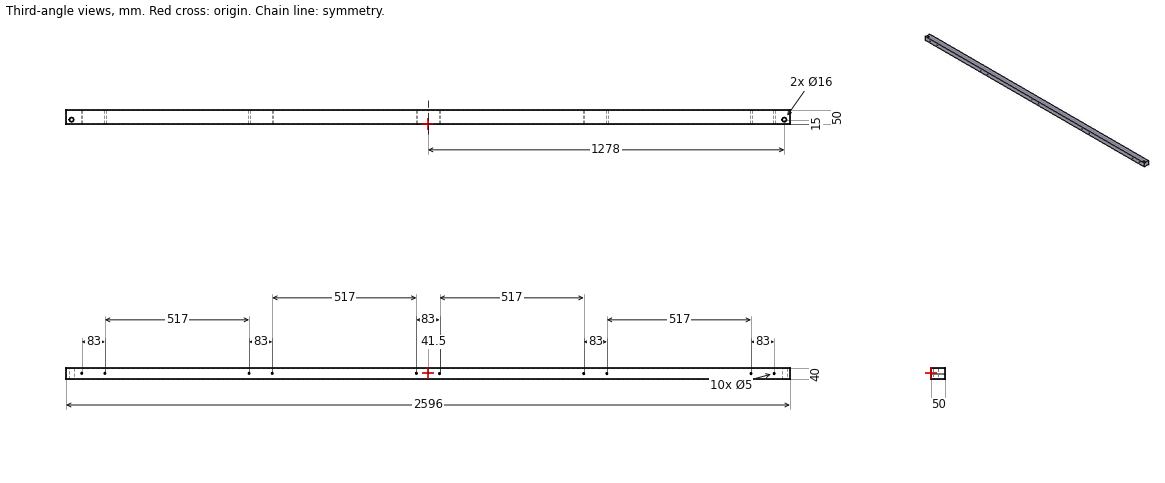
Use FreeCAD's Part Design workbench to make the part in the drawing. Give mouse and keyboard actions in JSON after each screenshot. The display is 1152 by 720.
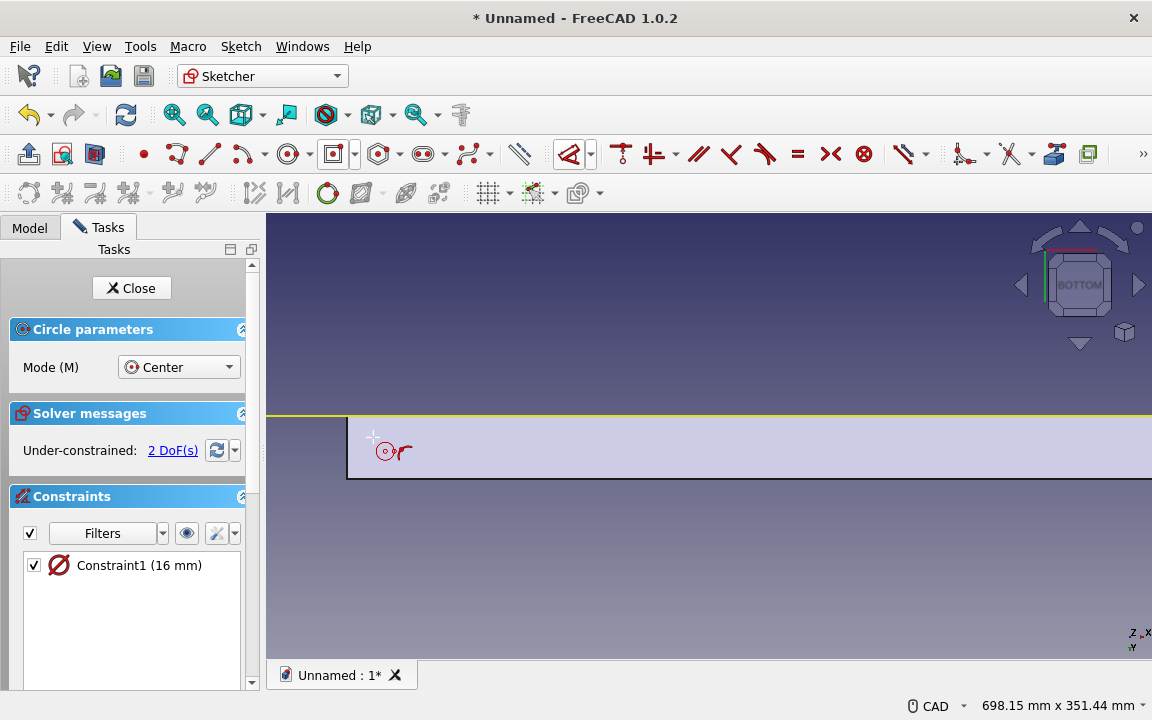
{"action": "left_click", "coordinate": [372, 435]}
{"action": "mouse_move", "coordinate": [379, 442]}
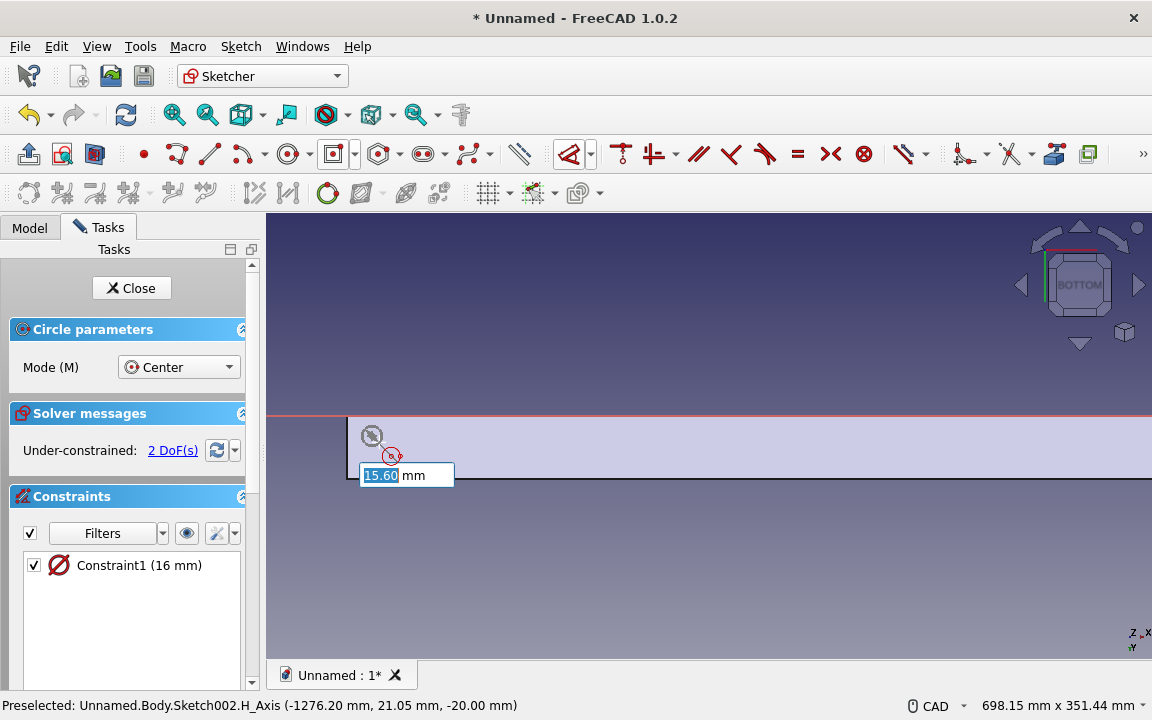
{"action": "type", "text": "16"}
{"action": "key", "text": "Return"}
{"action": "key", "text": "Escape"}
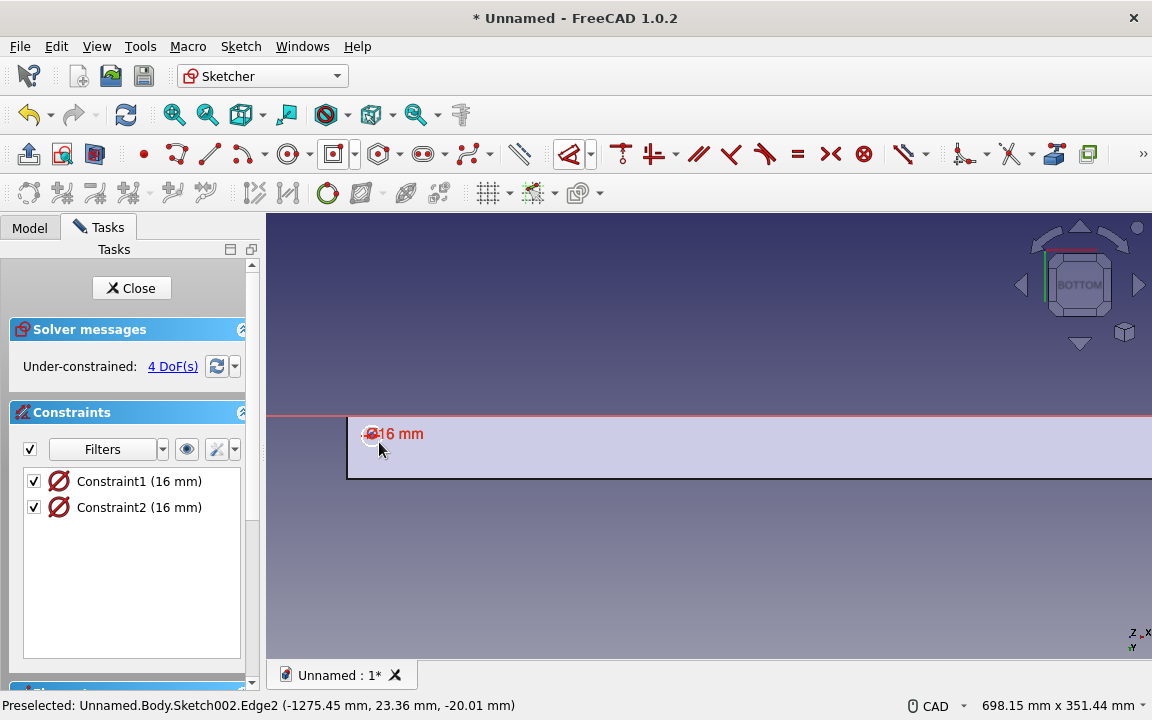
{"action": "scroll", "coordinate": [373, 437], "scroll_direction": "down", "scroll_amount": 9}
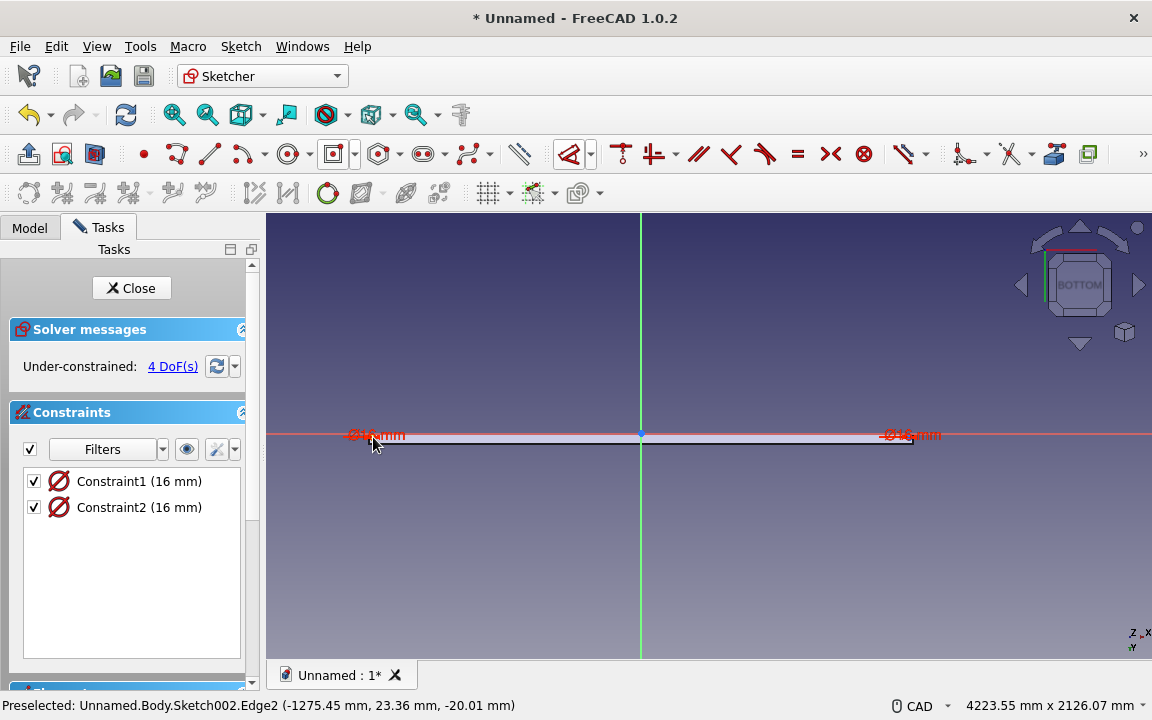
{"action": "left_click", "coordinate": [909, 437]}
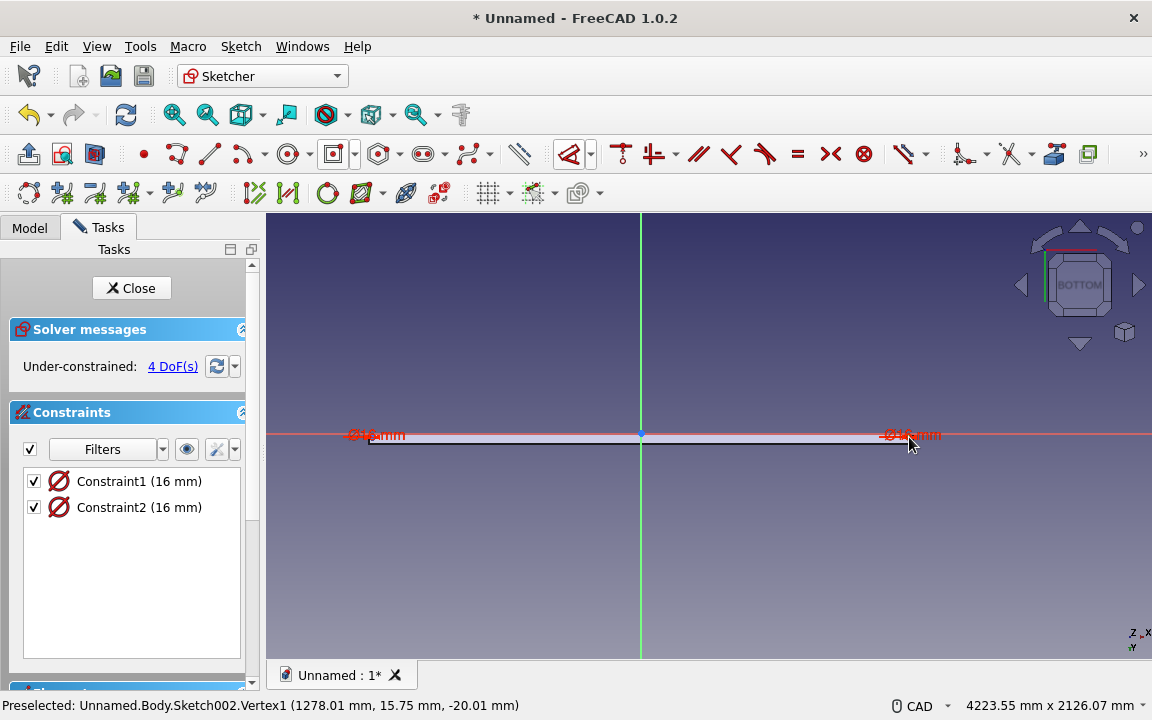
{"action": "left_click", "coordinate": [373, 437]}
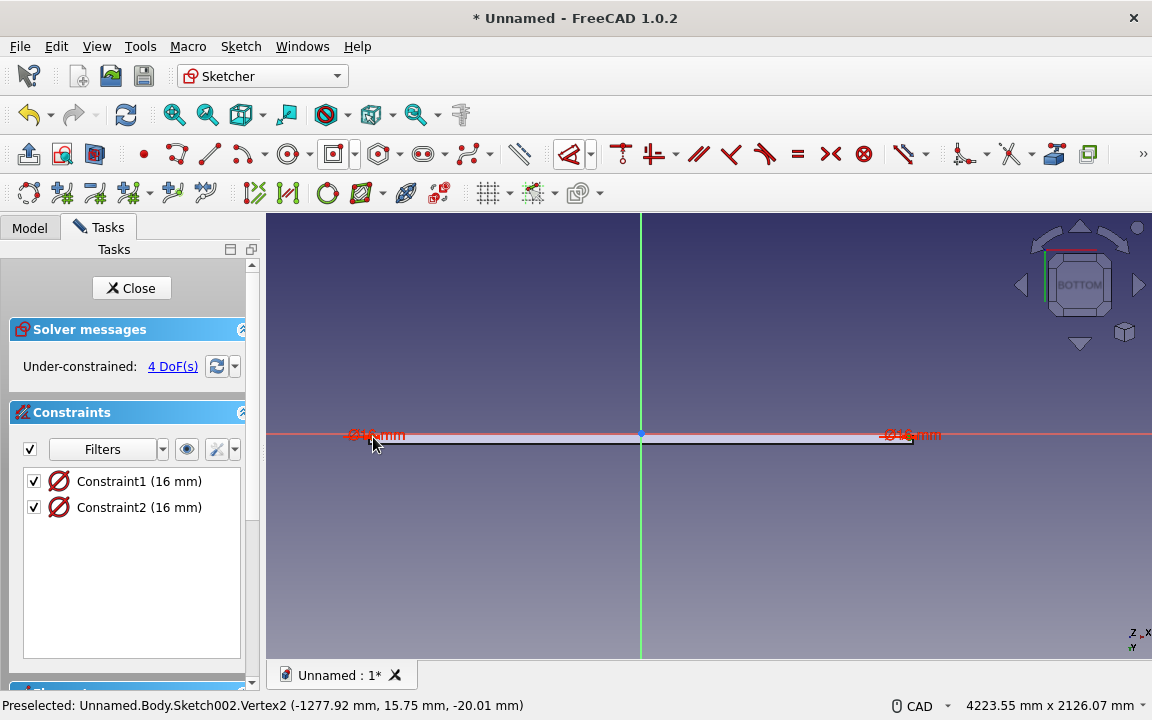
{"action": "left_click", "coordinate": [641, 603]}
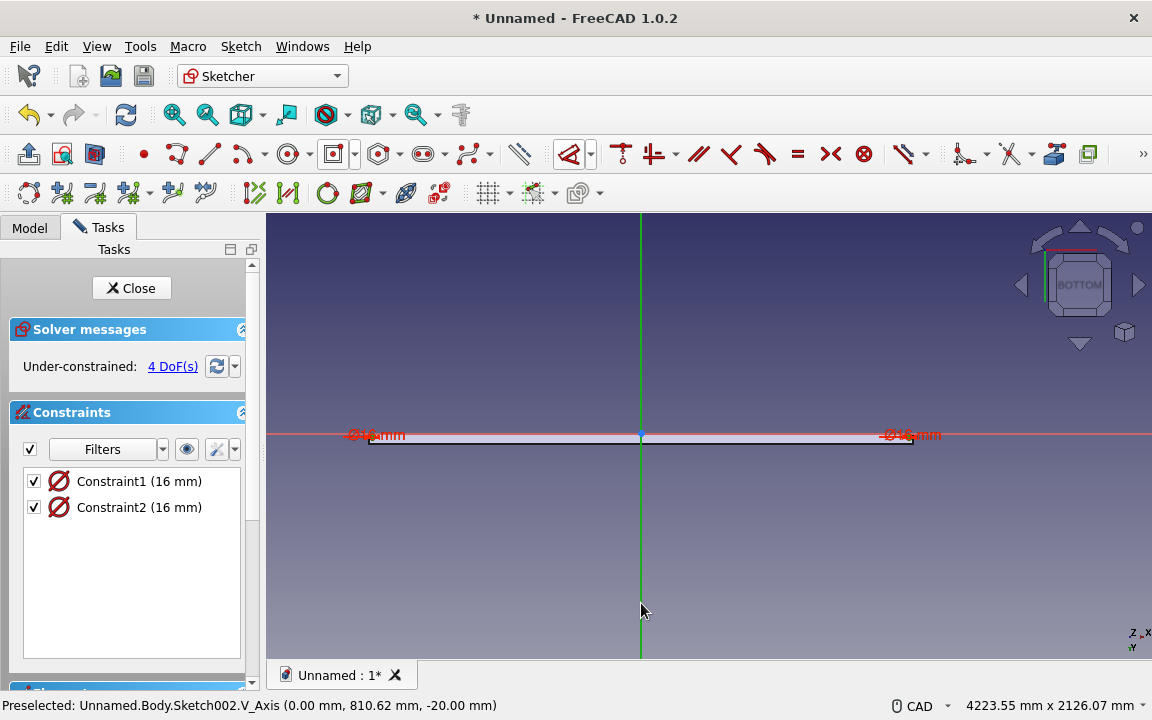
{"action": "left_click", "coordinate": [831, 154]}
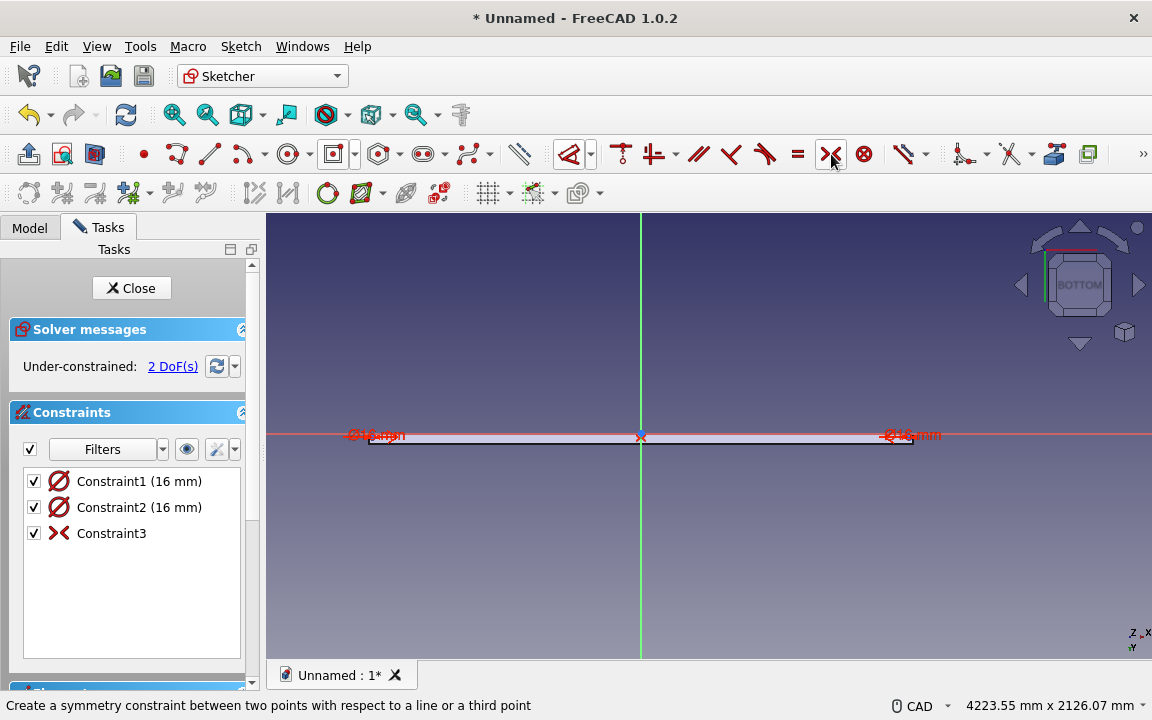
{"action": "scroll", "coordinate": [909, 437], "scroll_direction": "up", "scroll_amount": 13}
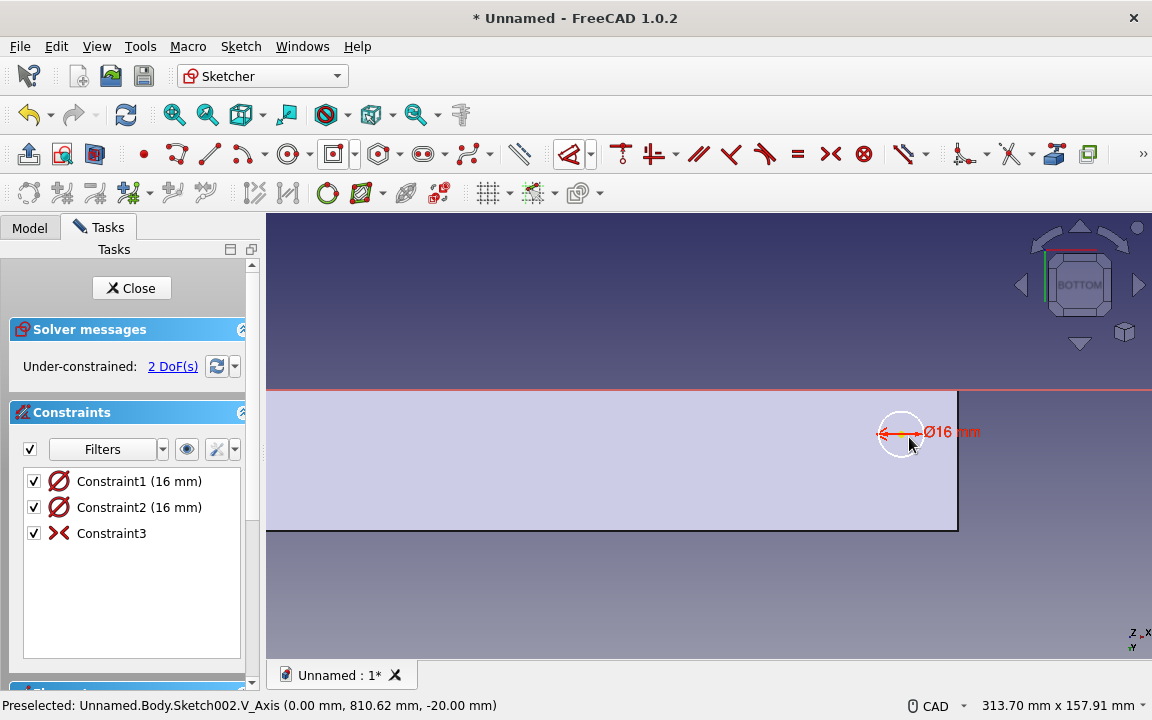
{"action": "left_click", "coordinate": [901, 434]}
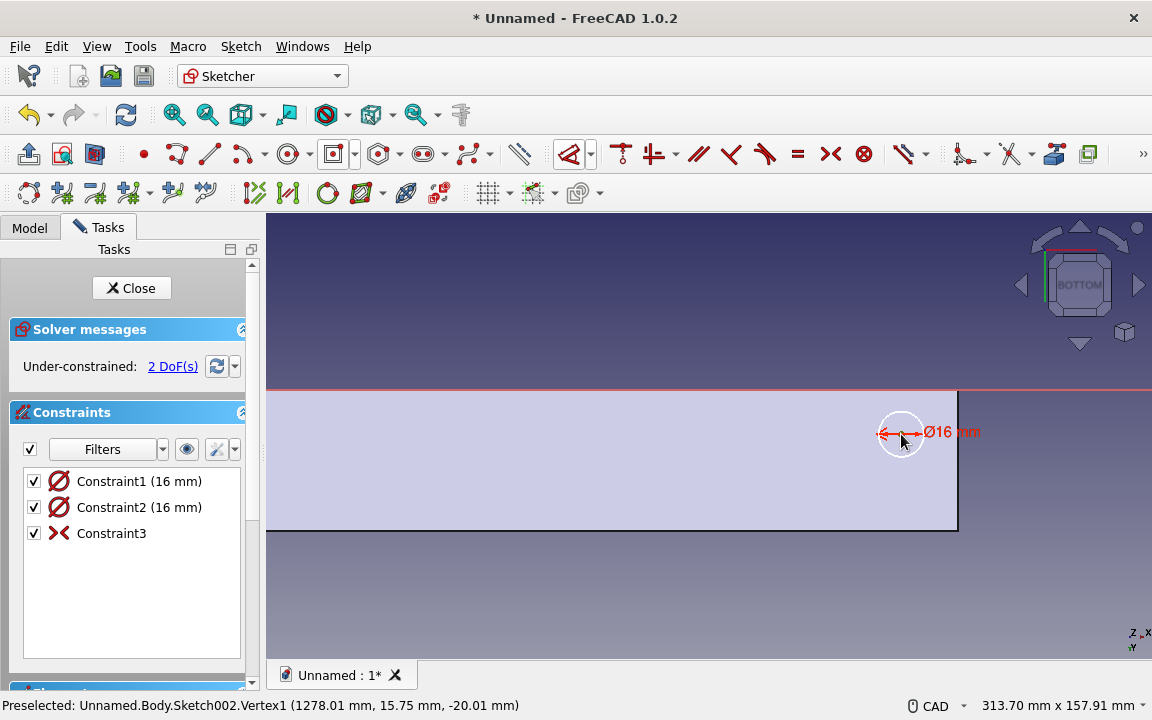
{"action": "left_click", "coordinate": [590, 154]}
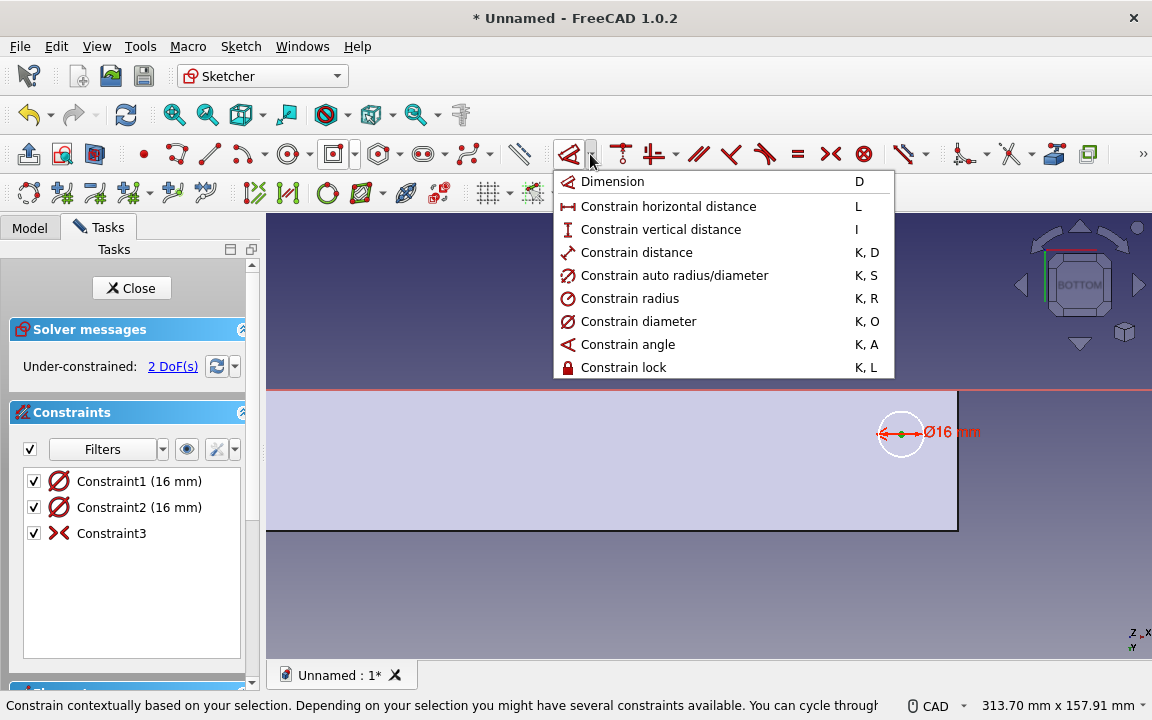
{"action": "left_click", "coordinate": [724, 230]}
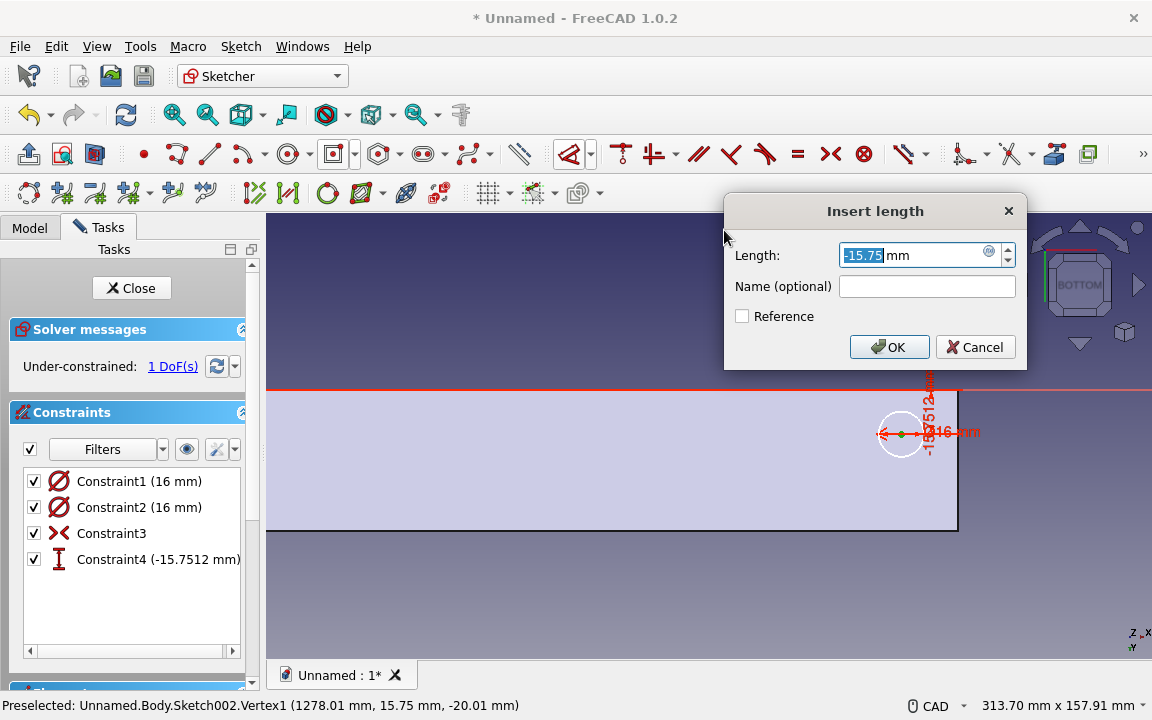
{"action": "type", "text": "-15"}
{"action": "key", "text": "Return"}